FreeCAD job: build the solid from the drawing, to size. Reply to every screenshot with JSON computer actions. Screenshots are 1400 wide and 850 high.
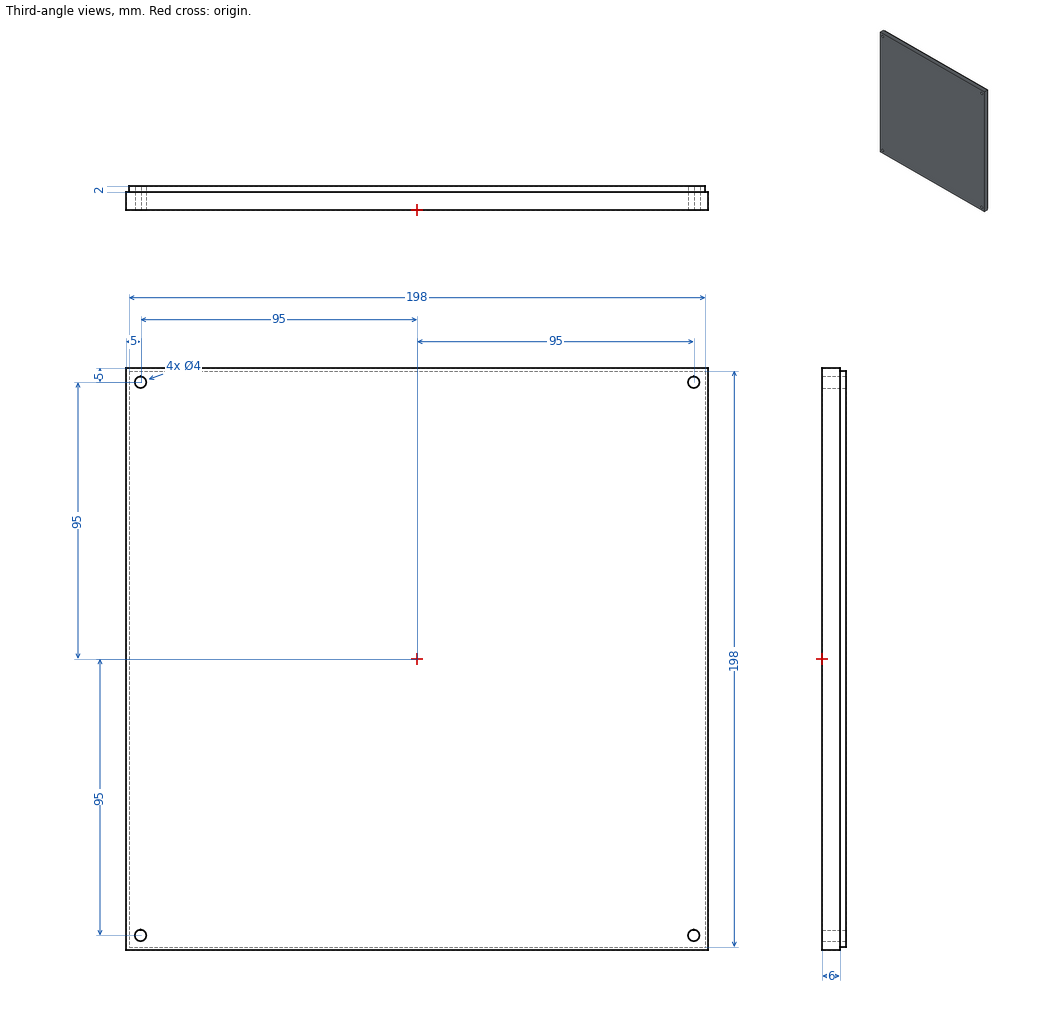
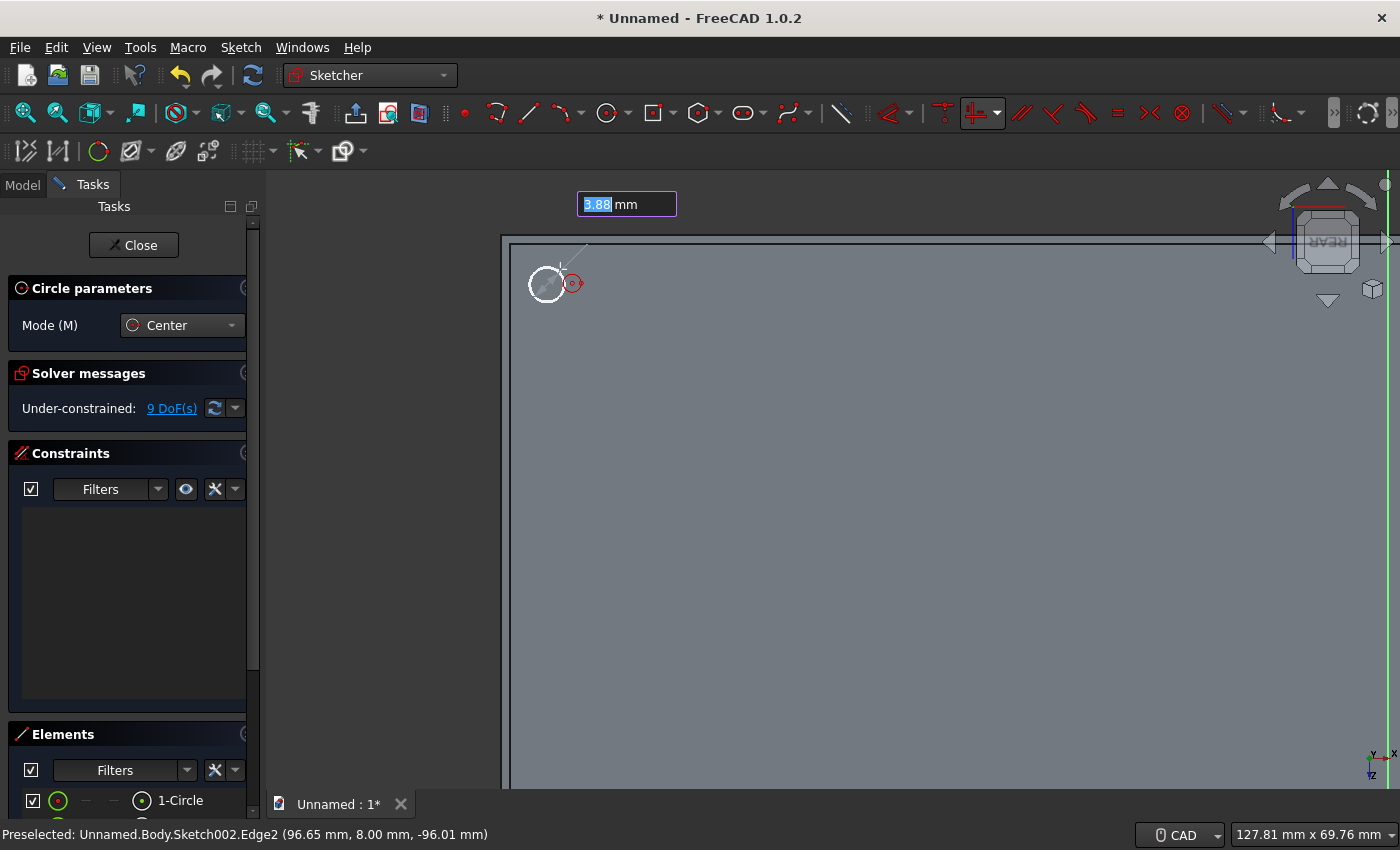
{"action": "left_click", "coordinate": [558, 267]}
{"action": "key", "text": "Escape"}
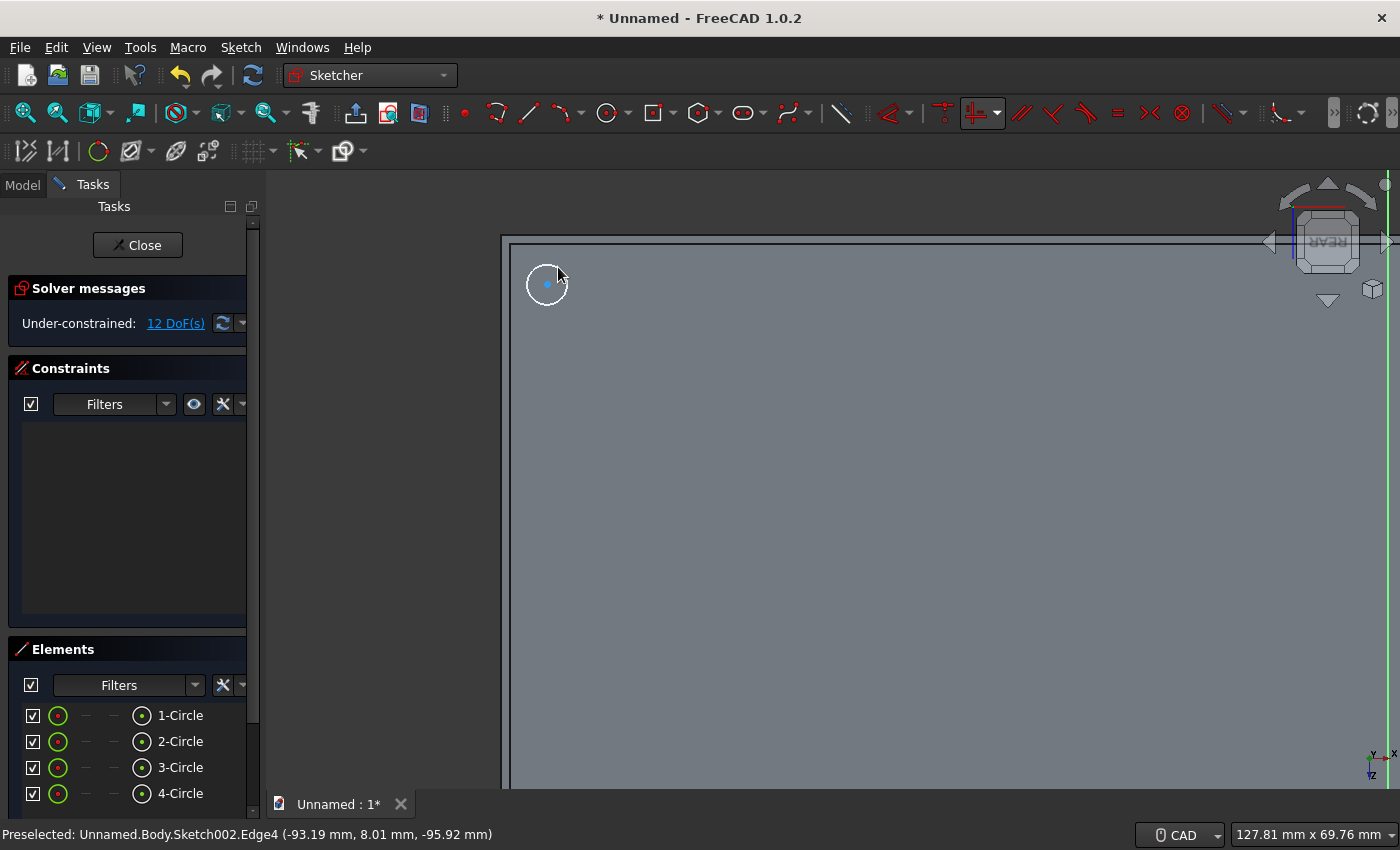
{"action": "scroll", "coordinate": [560, 269], "scroll_direction": "down", "scroll_amount": 7}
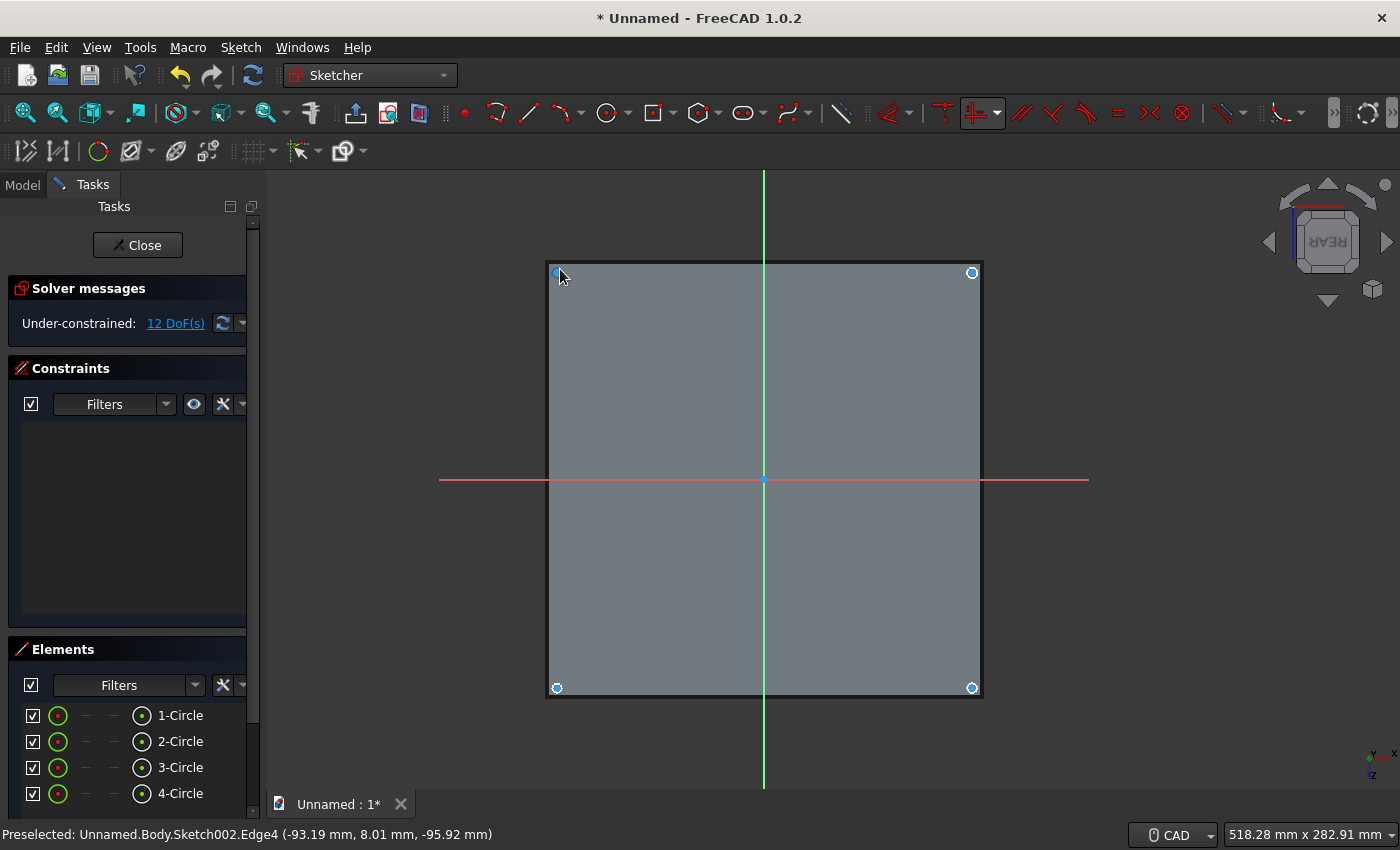
{"action": "scroll", "coordinate": [560, 685], "scroll_direction": "up", "scroll_amount": 6}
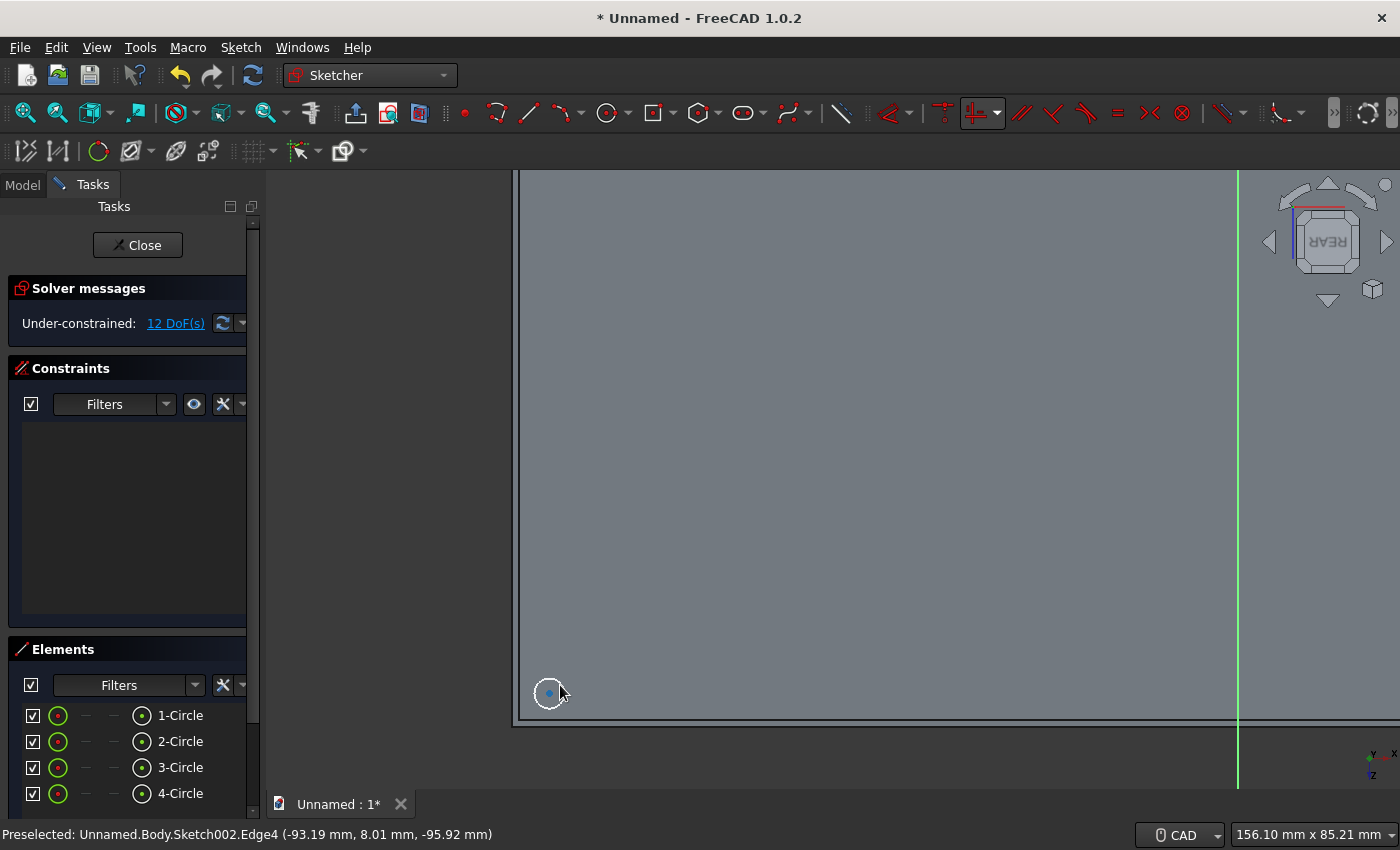
{"action": "left_click", "coordinate": [560, 683]}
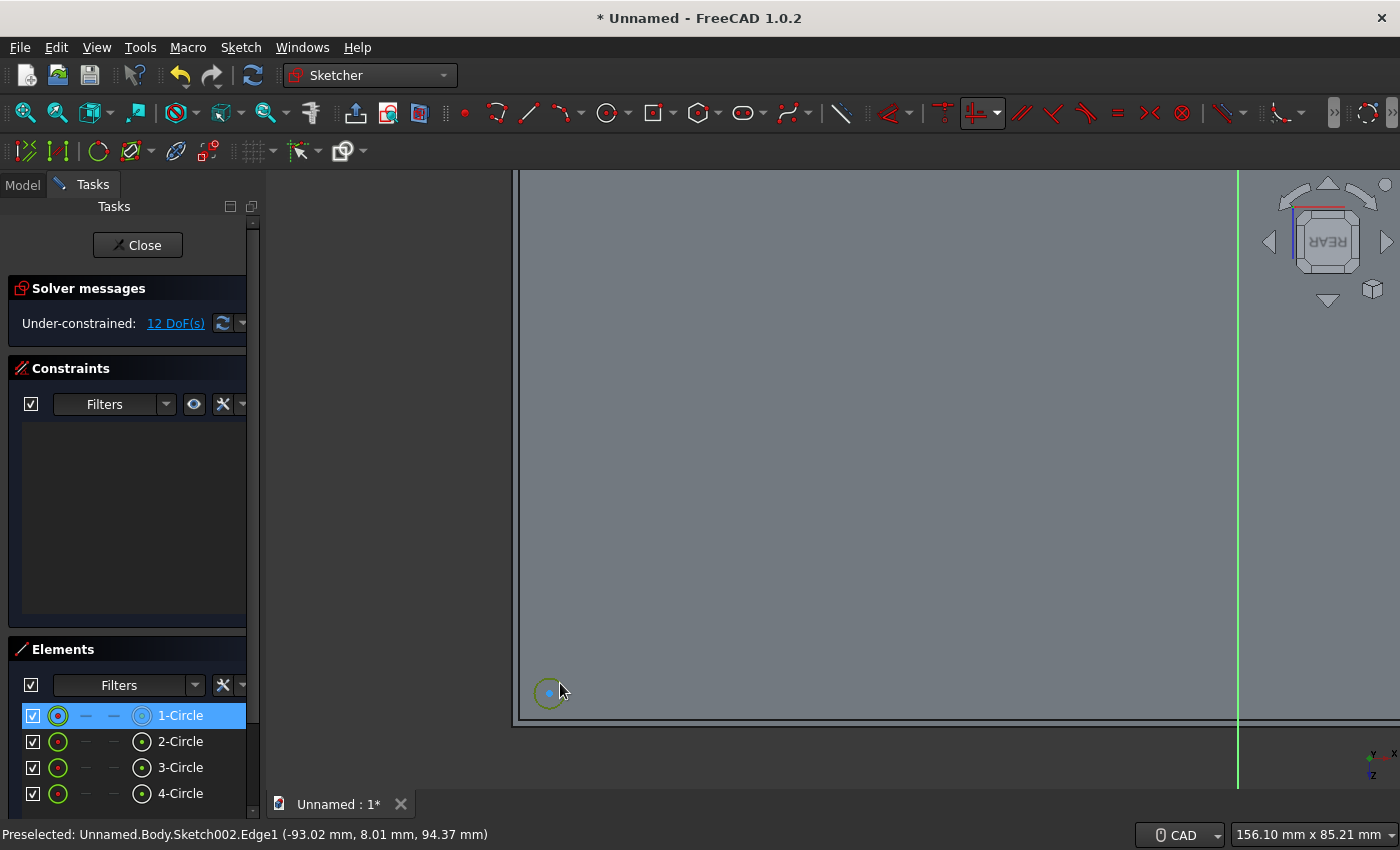
{"action": "scroll", "coordinate": [560, 686], "scroll_direction": "down", "scroll_amount": 6}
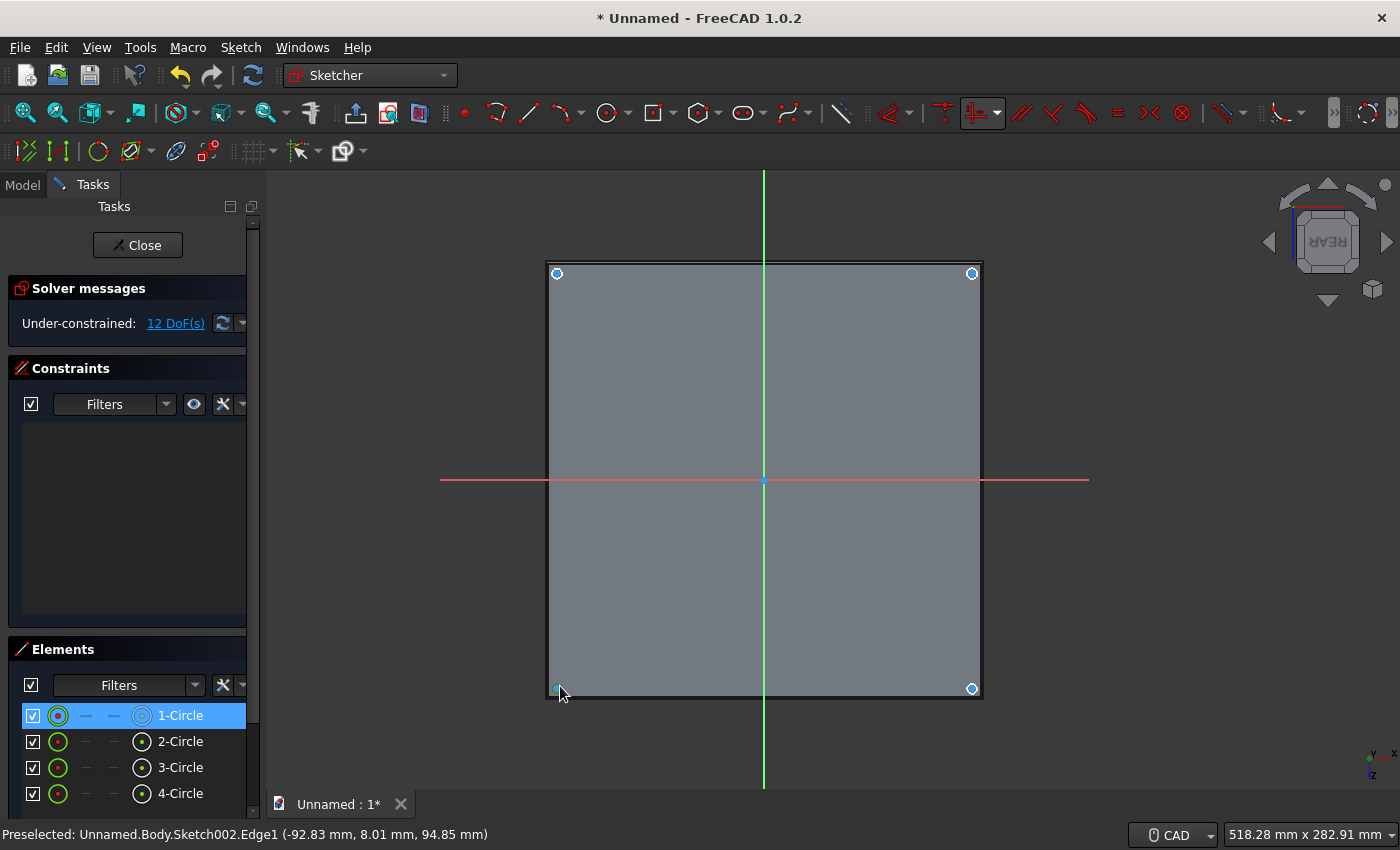
{"action": "scroll", "coordinate": [976, 685], "scroll_direction": "up", "scroll_amount": 6}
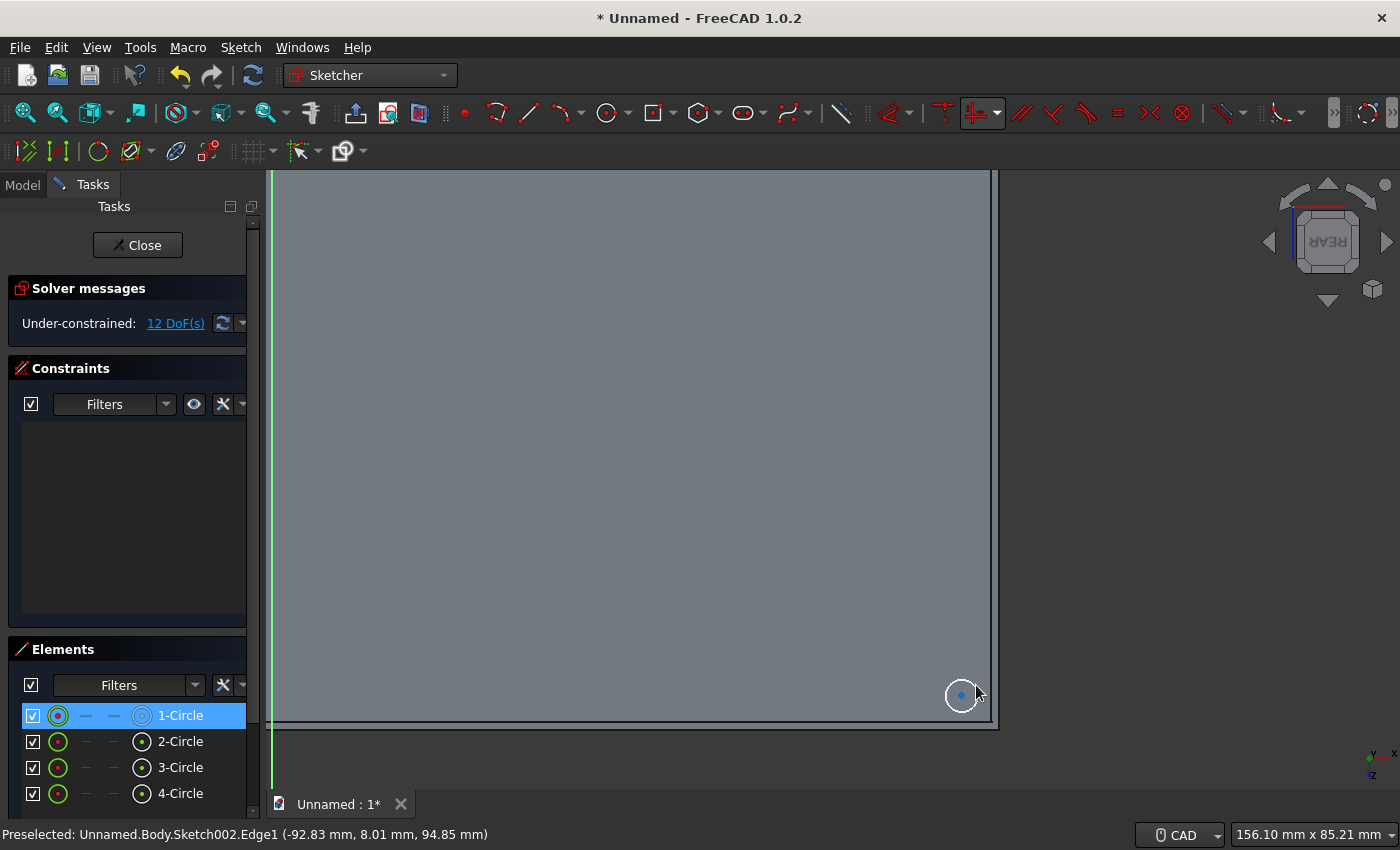
{"action": "left_click", "coordinate": [973, 684]}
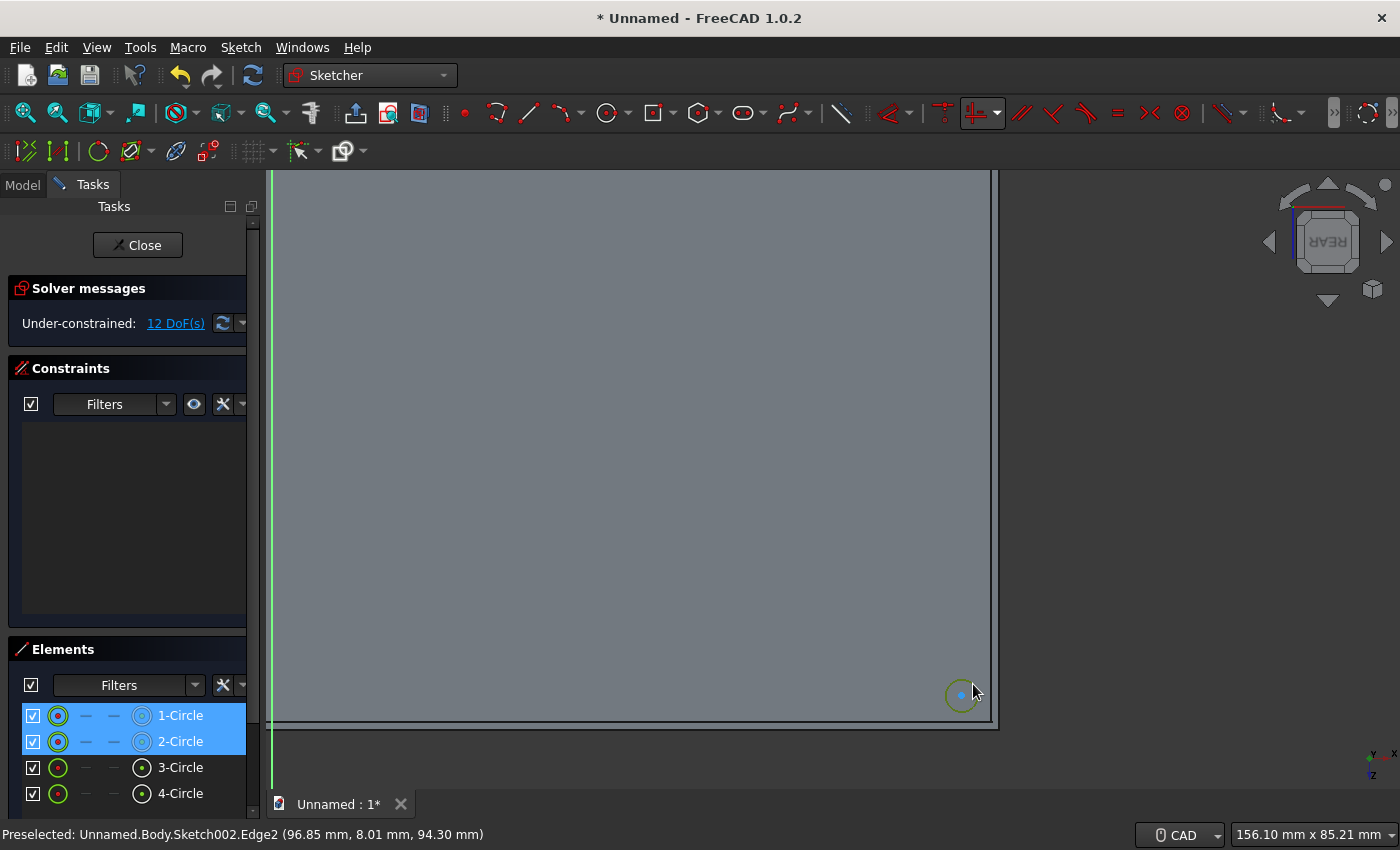
{"action": "scroll", "coordinate": [977, 685], "scroll_direction": "down", "scroll_amount": 6}